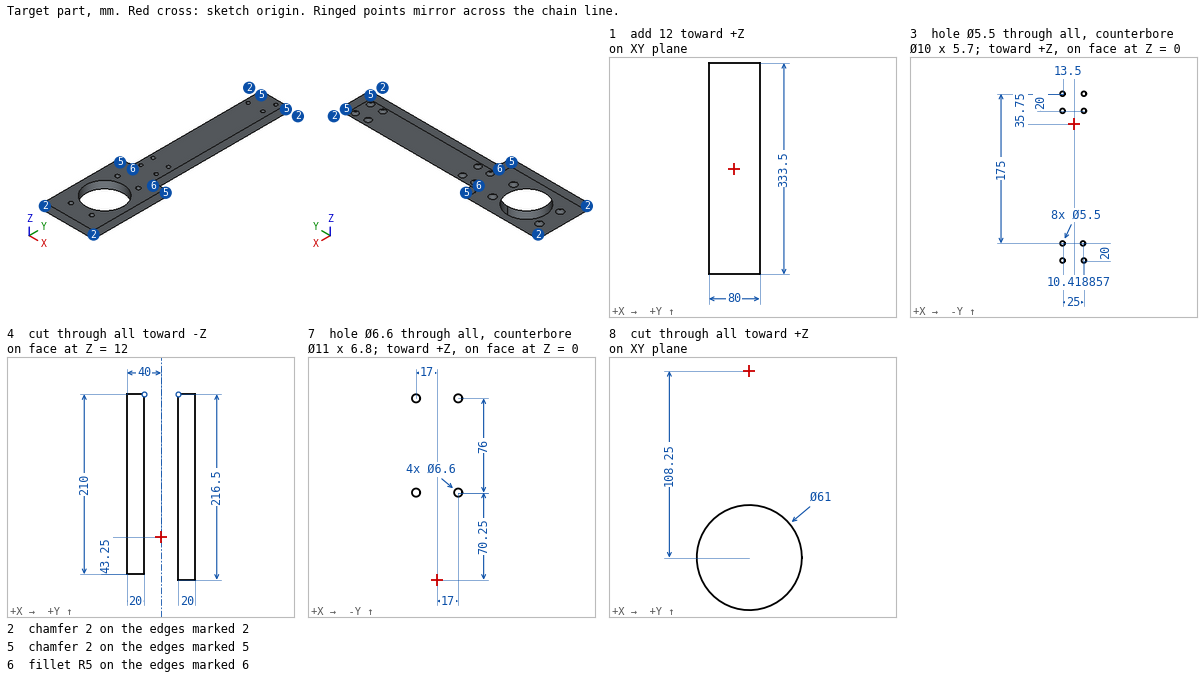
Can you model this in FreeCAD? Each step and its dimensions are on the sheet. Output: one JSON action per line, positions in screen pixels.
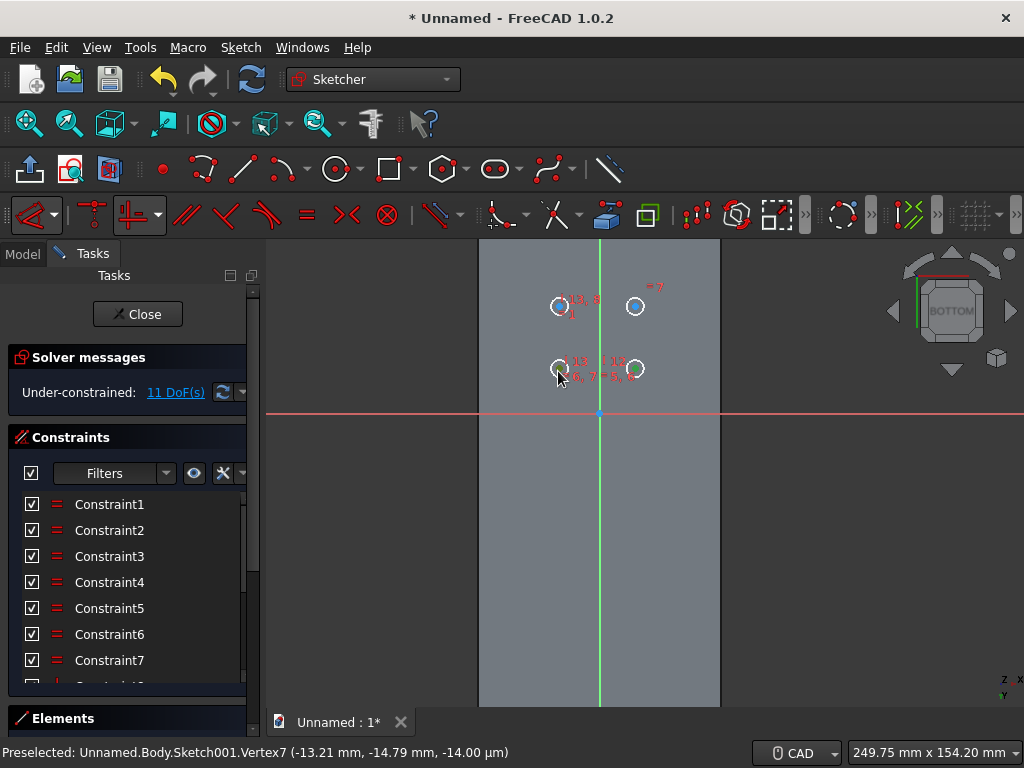
{"action": "left_click", "coordinate": [160, 216]}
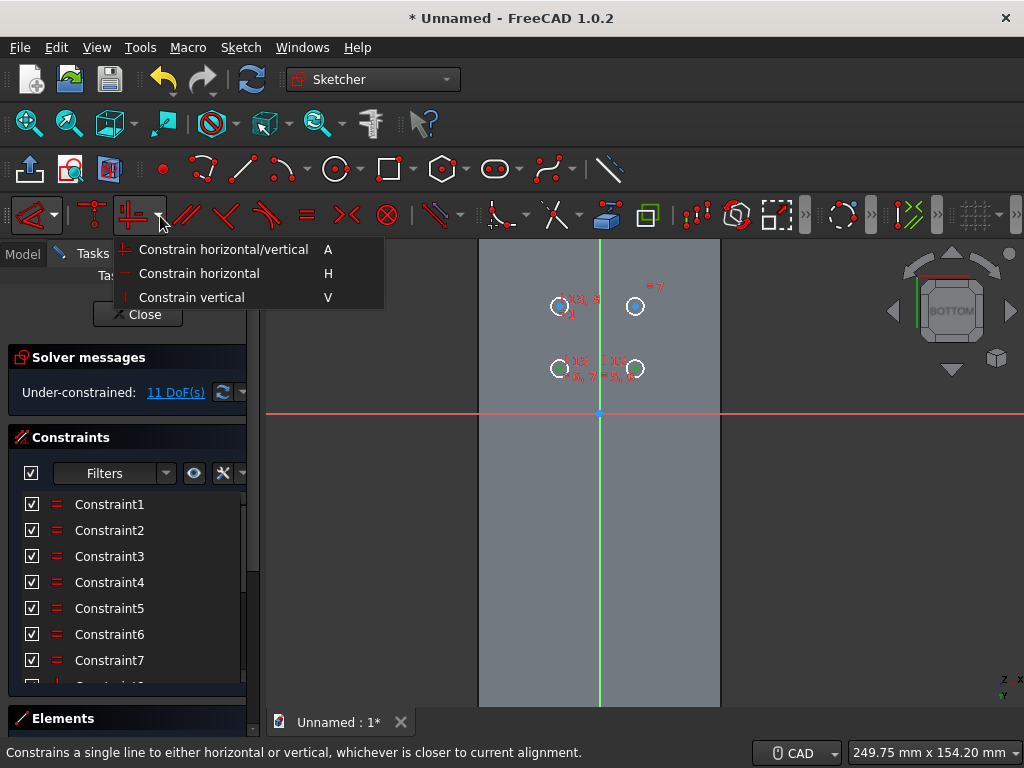
{"action": "left_click", "coordinate": [249, 273]}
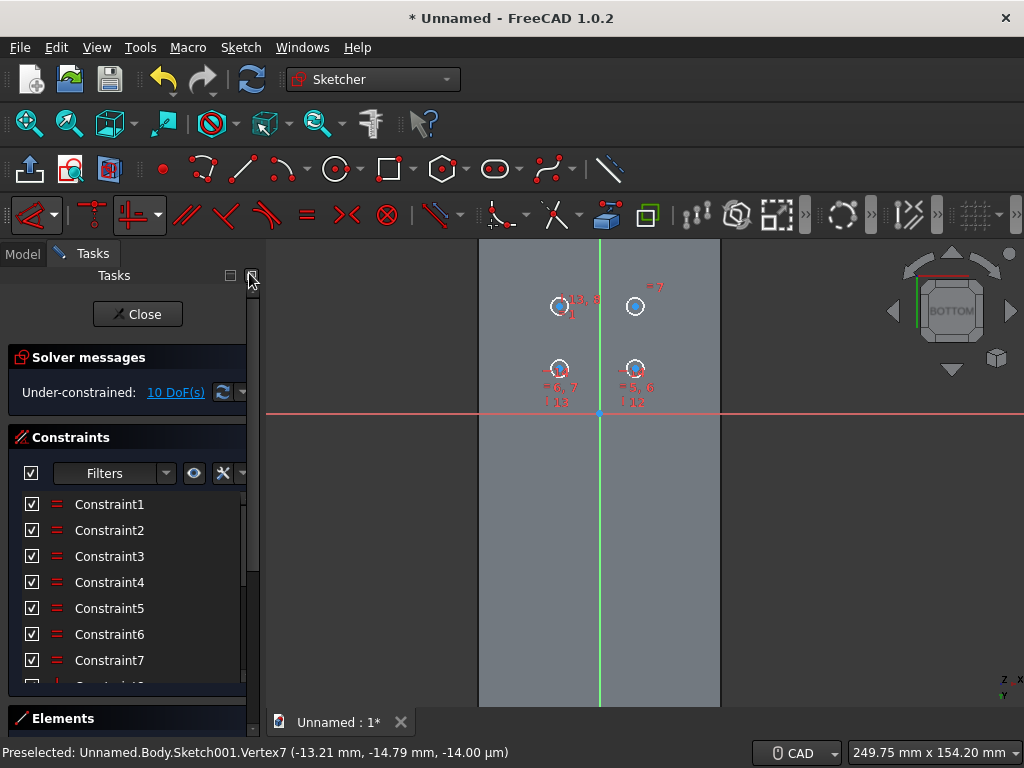
{"action": "left_click", "coordinate": [635, 369]}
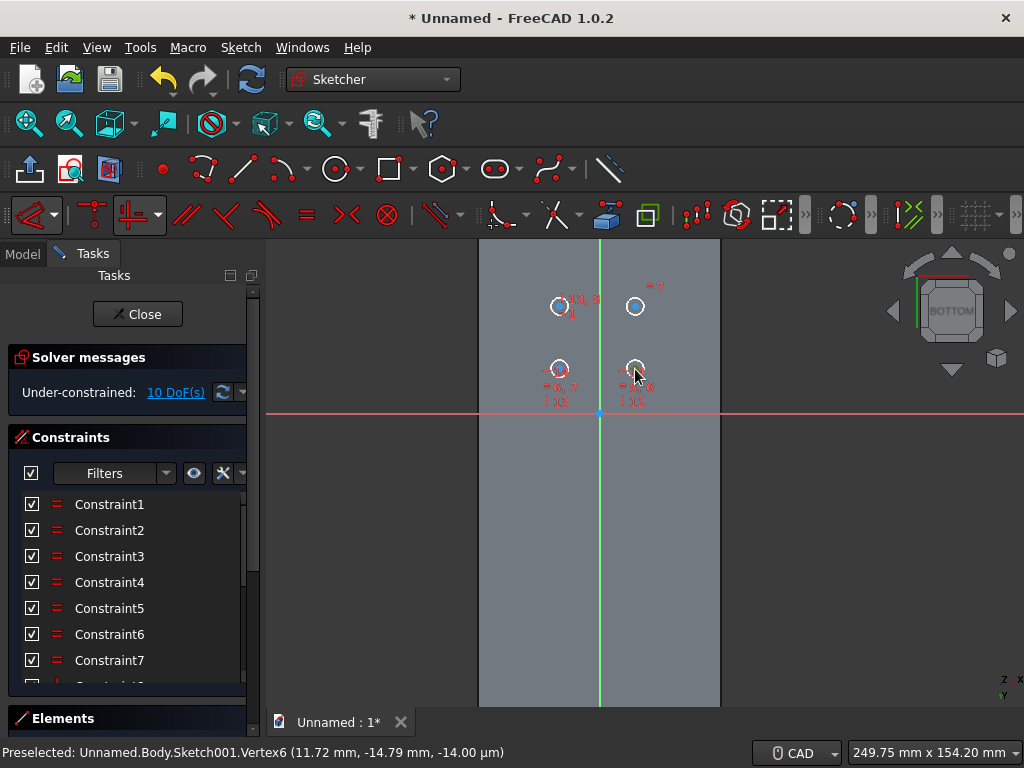
{"action": "left_click", "coordinate": [635, 306]}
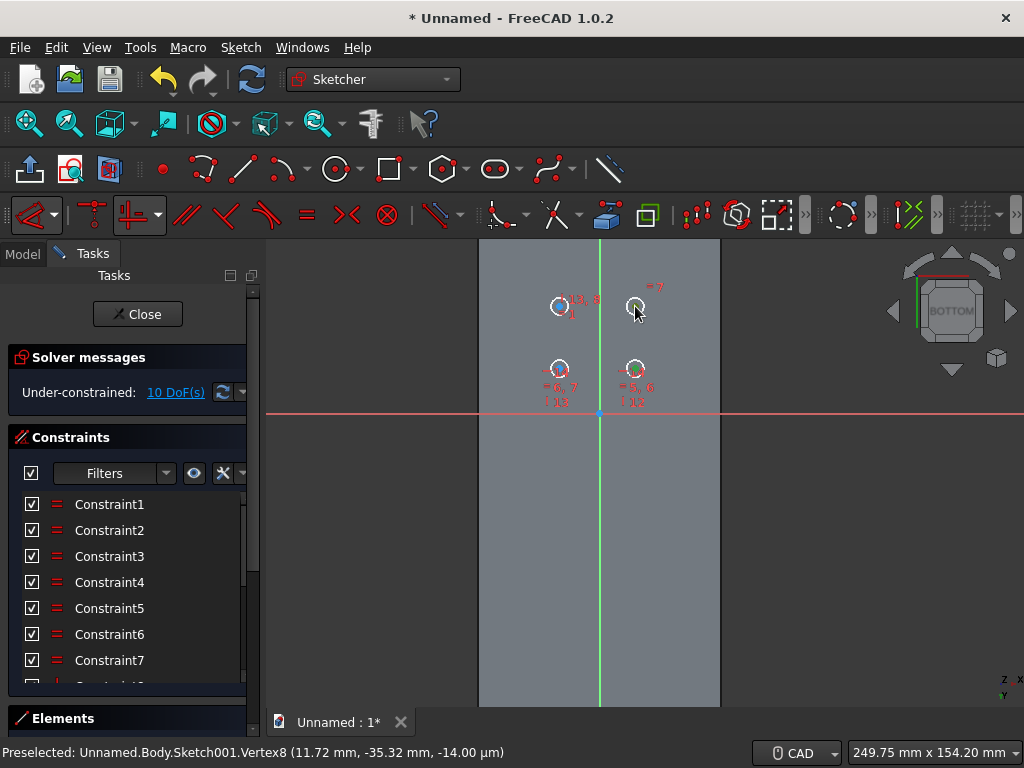
{"action": "key", "text": "v"}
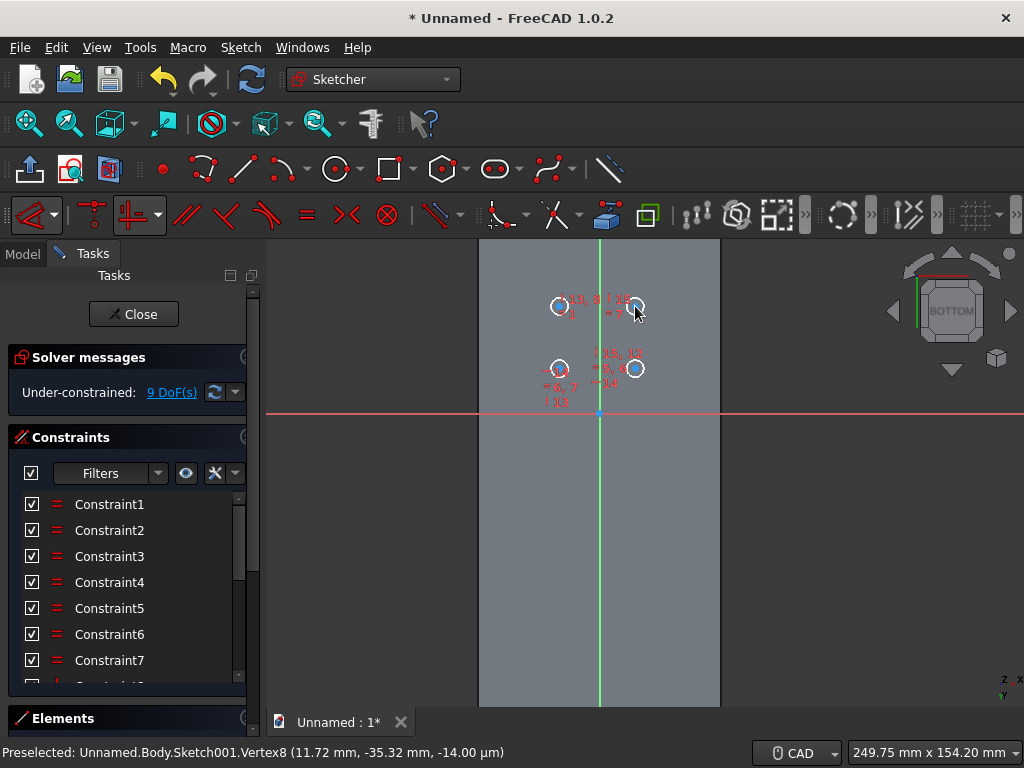
{"action": "left_click", "coordinate": [560, 306]}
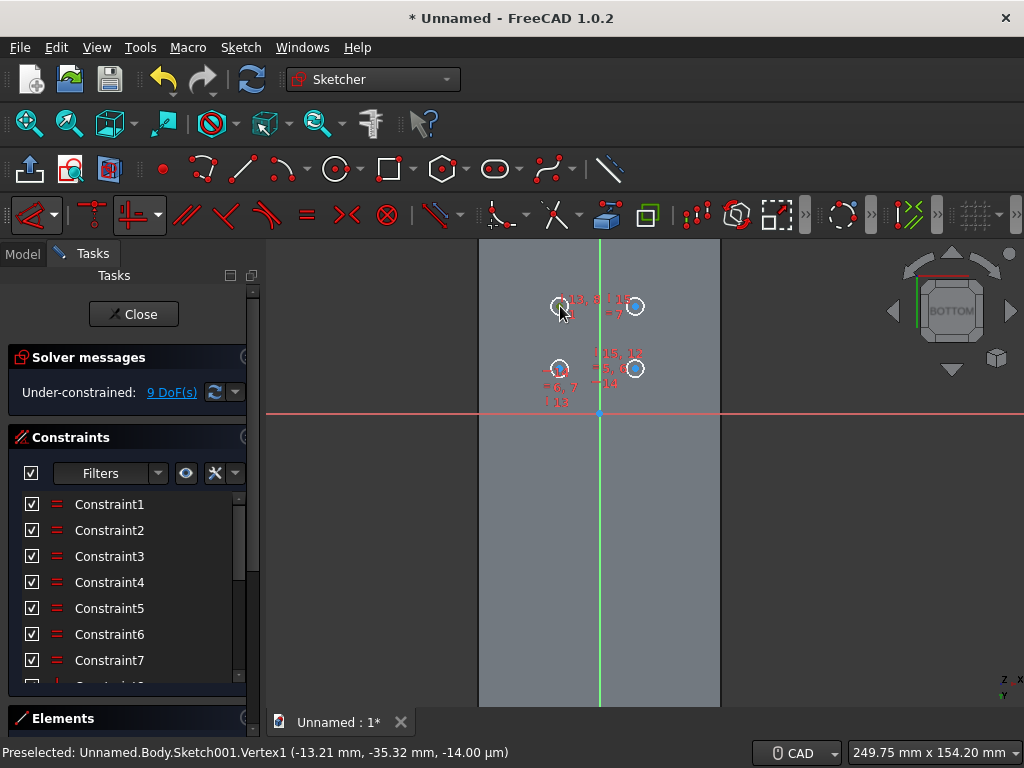
{"action": "left_click", "coordinate": [635, 306]}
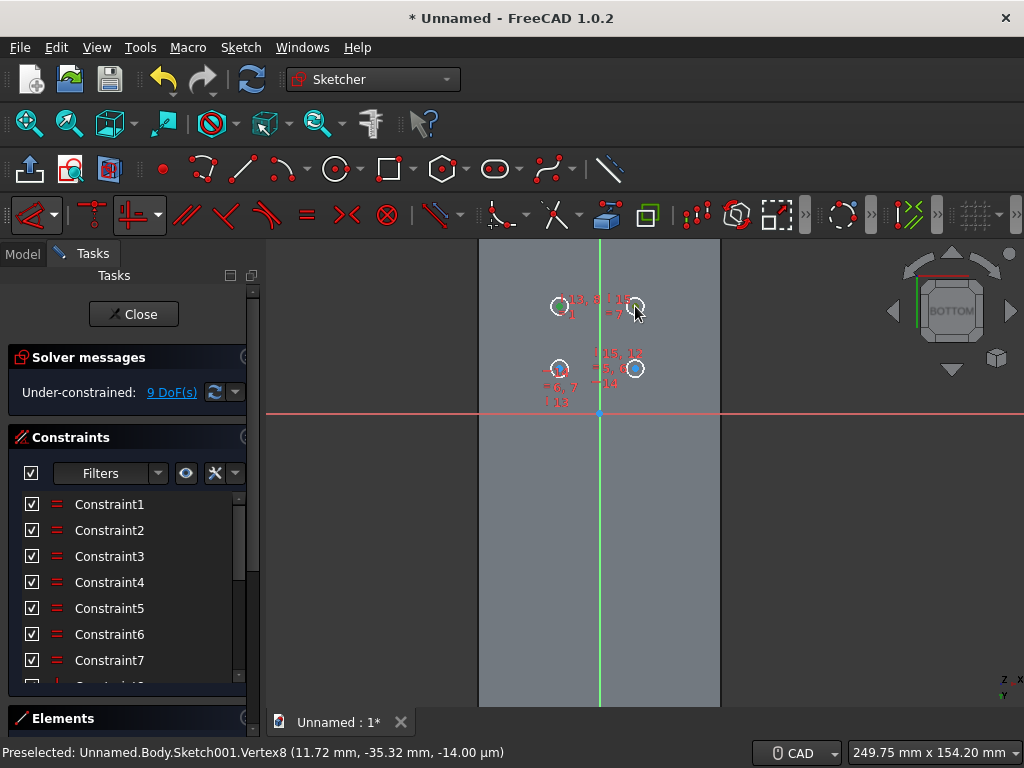
{"action": "key", "text": "h"}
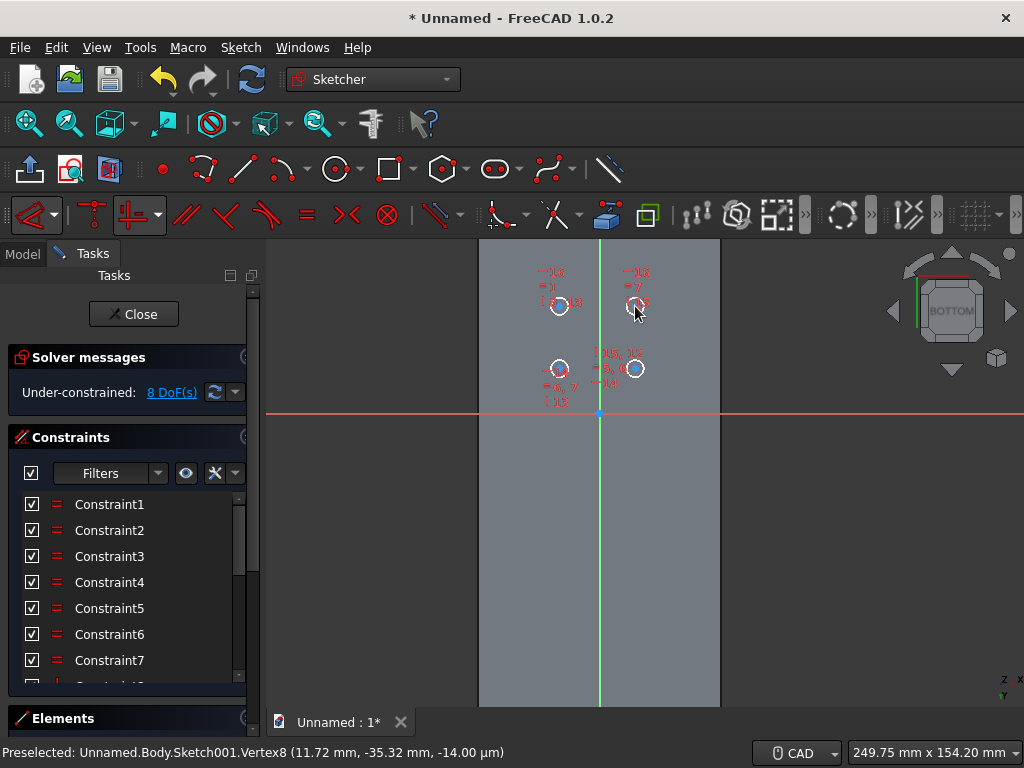
{"action": "key", "text": "d"}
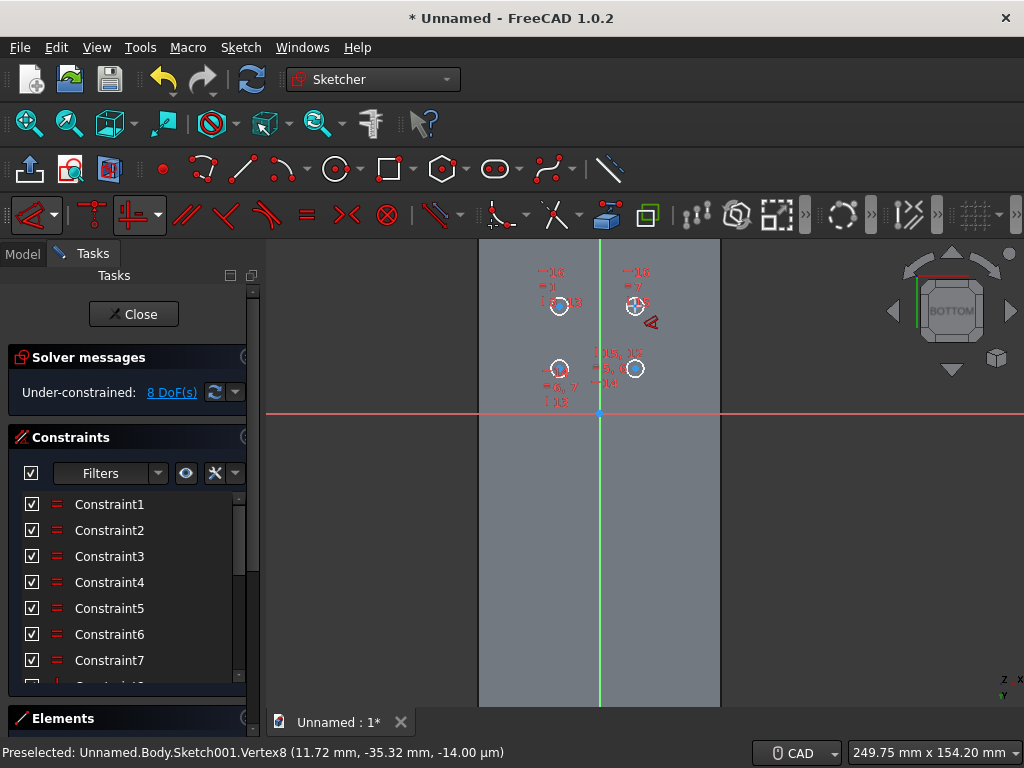
{"action": "scroll", "coordinate": [566, 300], "scroll_direction": "up", "scroll_amount": 5}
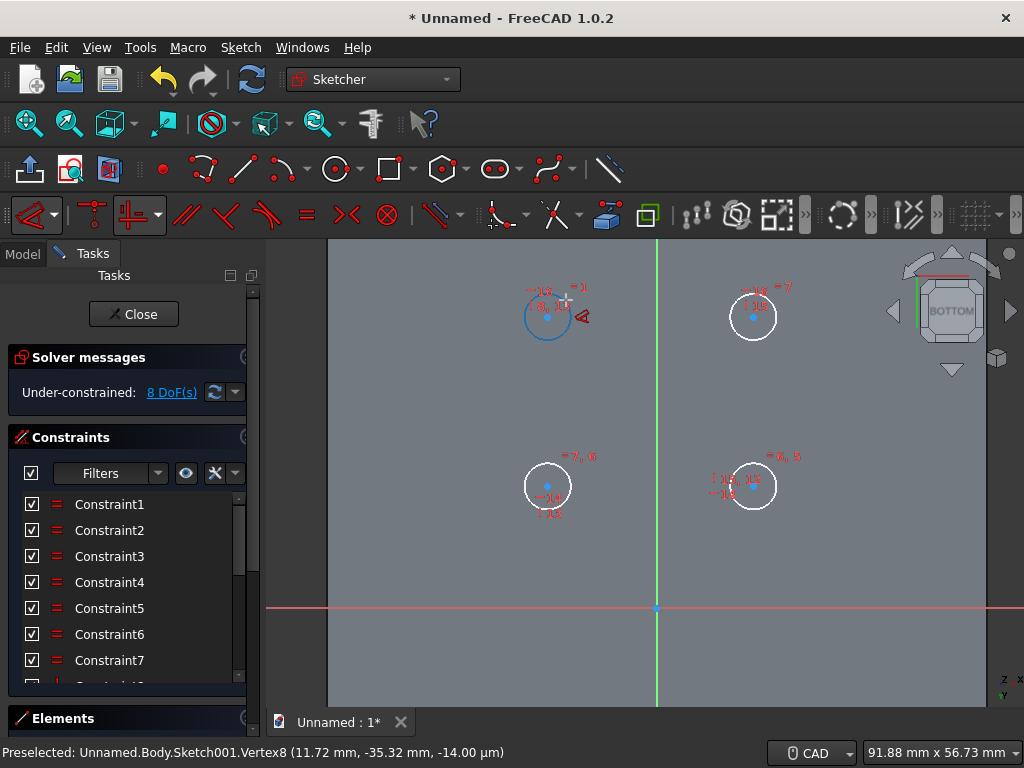
{"action": "left_click", "coordinate": [564, 301]}
{"action": "left_click", "coordinate": [587, 279]}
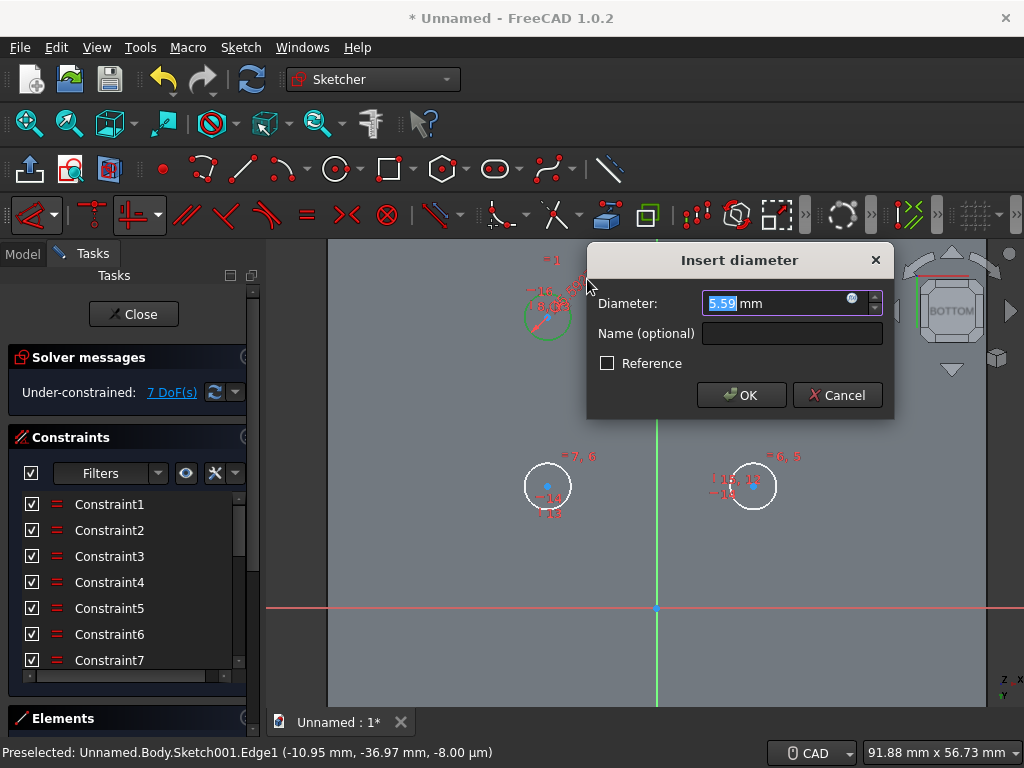
{"action": "type", "text": "5.5"}
{"action": "key", "text": "Return"}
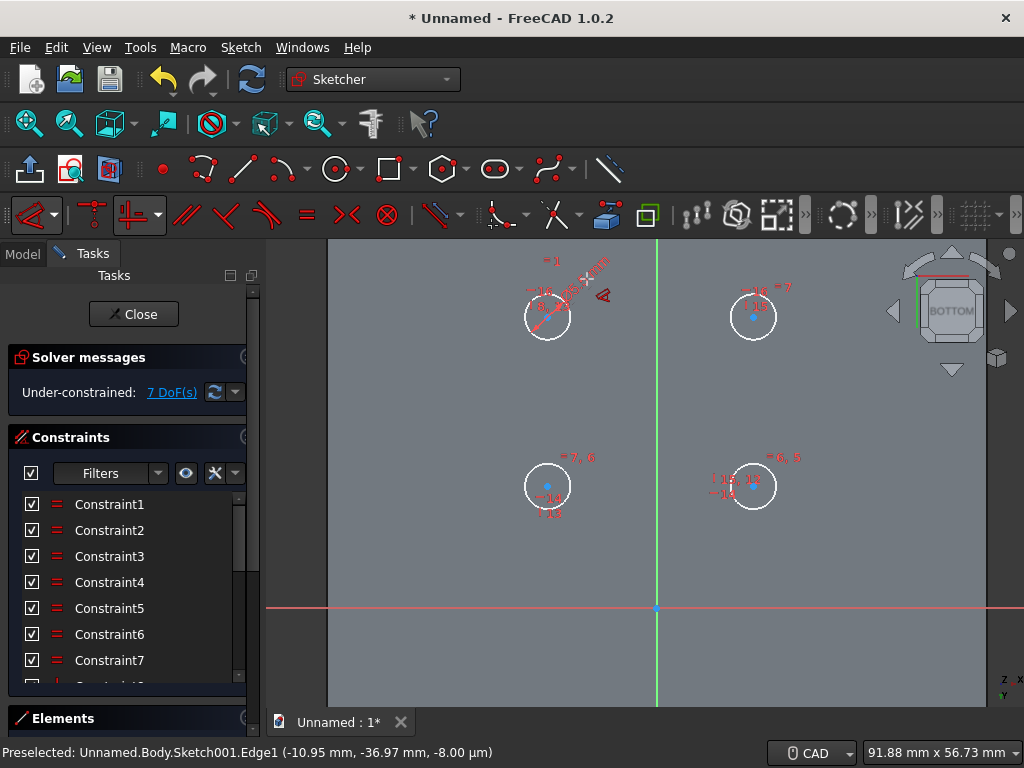
{"action": "scroll", "coordinate": [562, 345], "scroll_direction": "down", "scroll_amount": 9}